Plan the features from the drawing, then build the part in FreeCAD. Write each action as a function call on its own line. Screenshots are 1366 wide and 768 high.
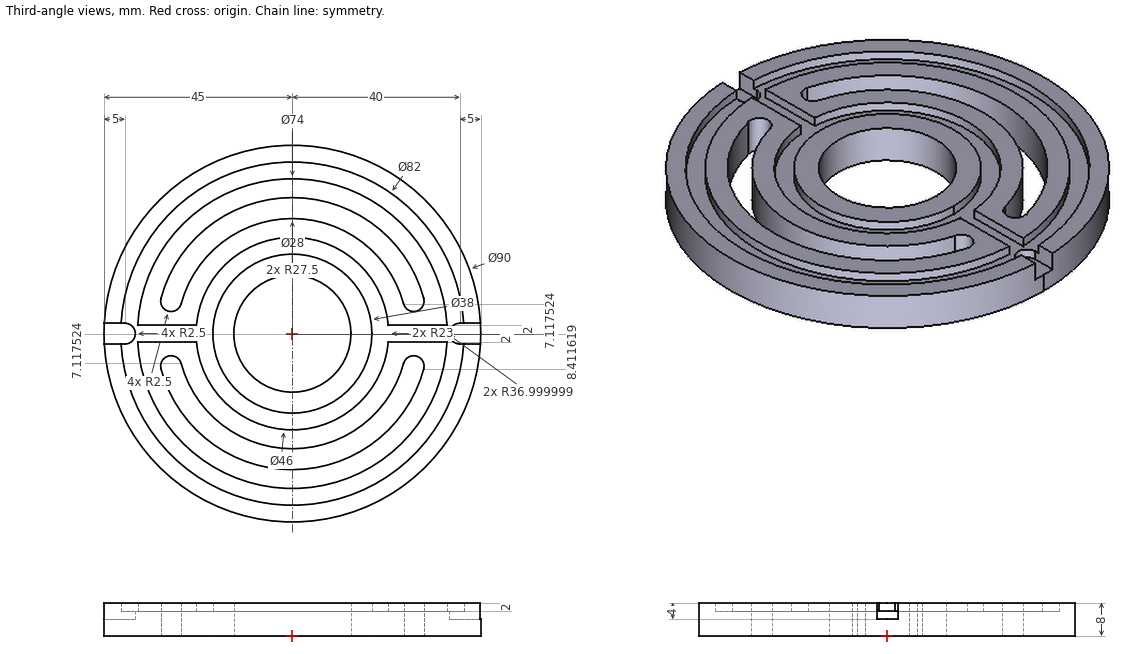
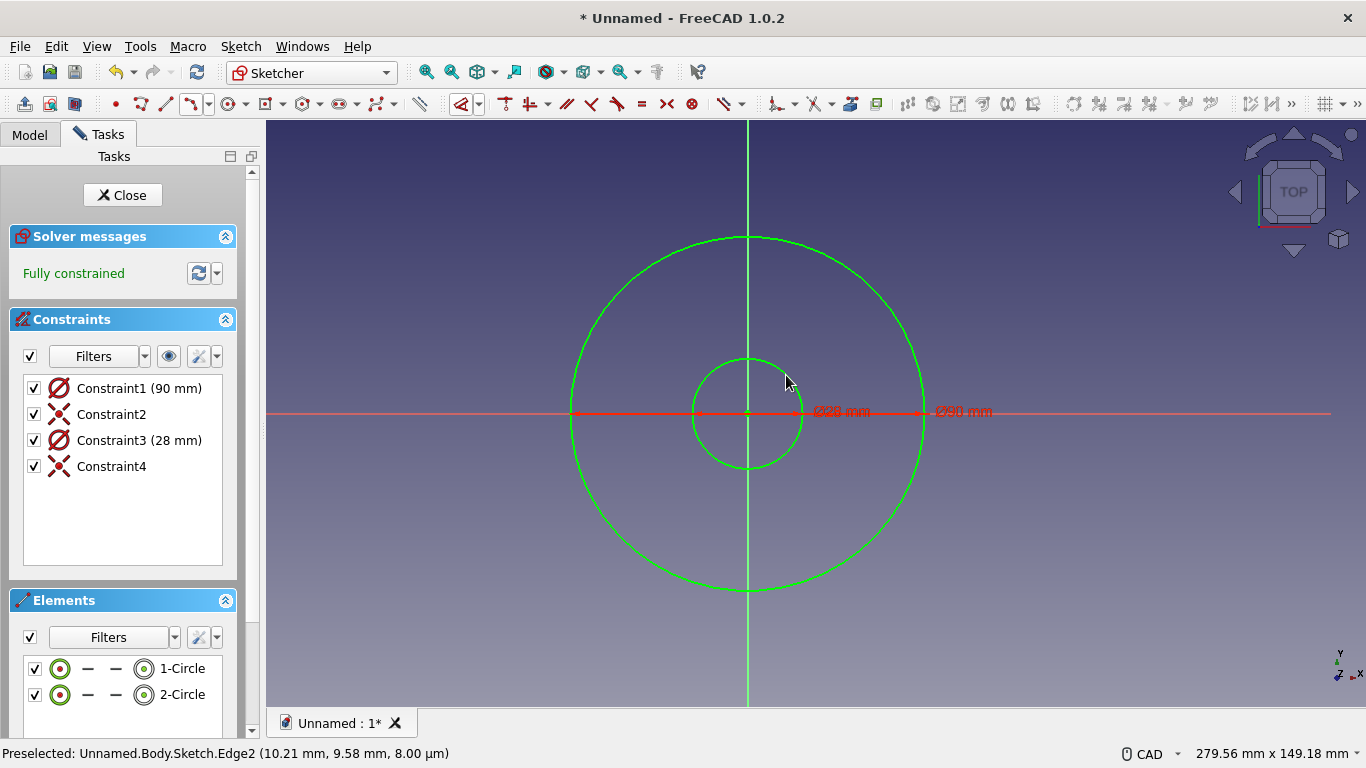
click(123, 195)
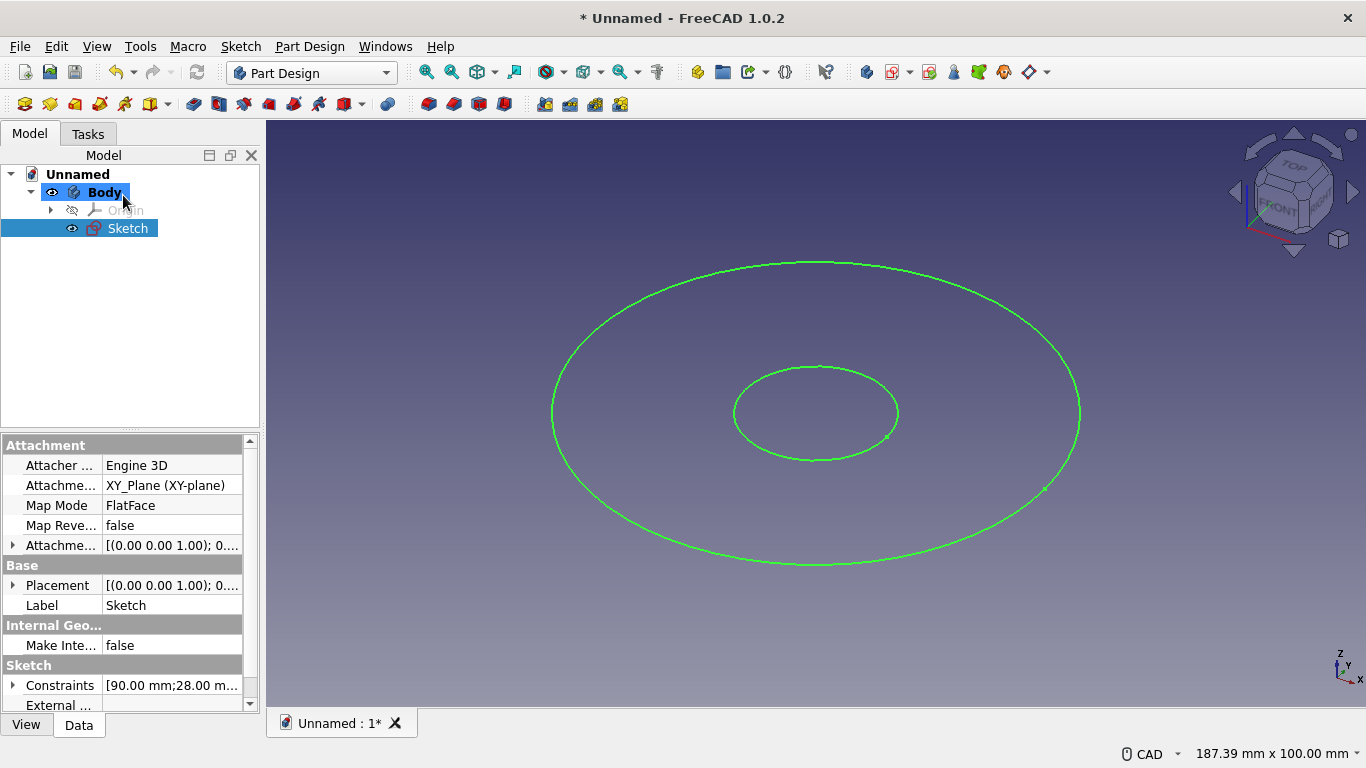
click(25, 104)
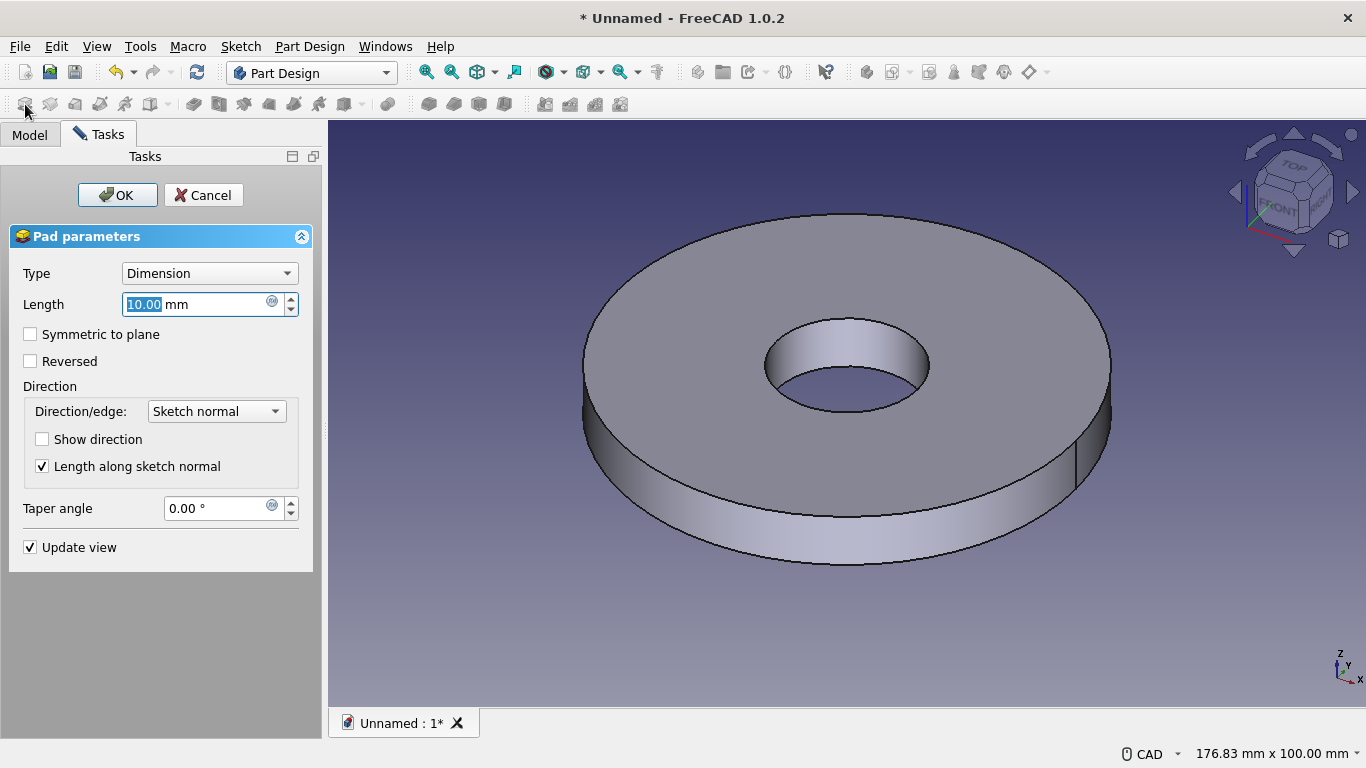
text(8)
key(Tab)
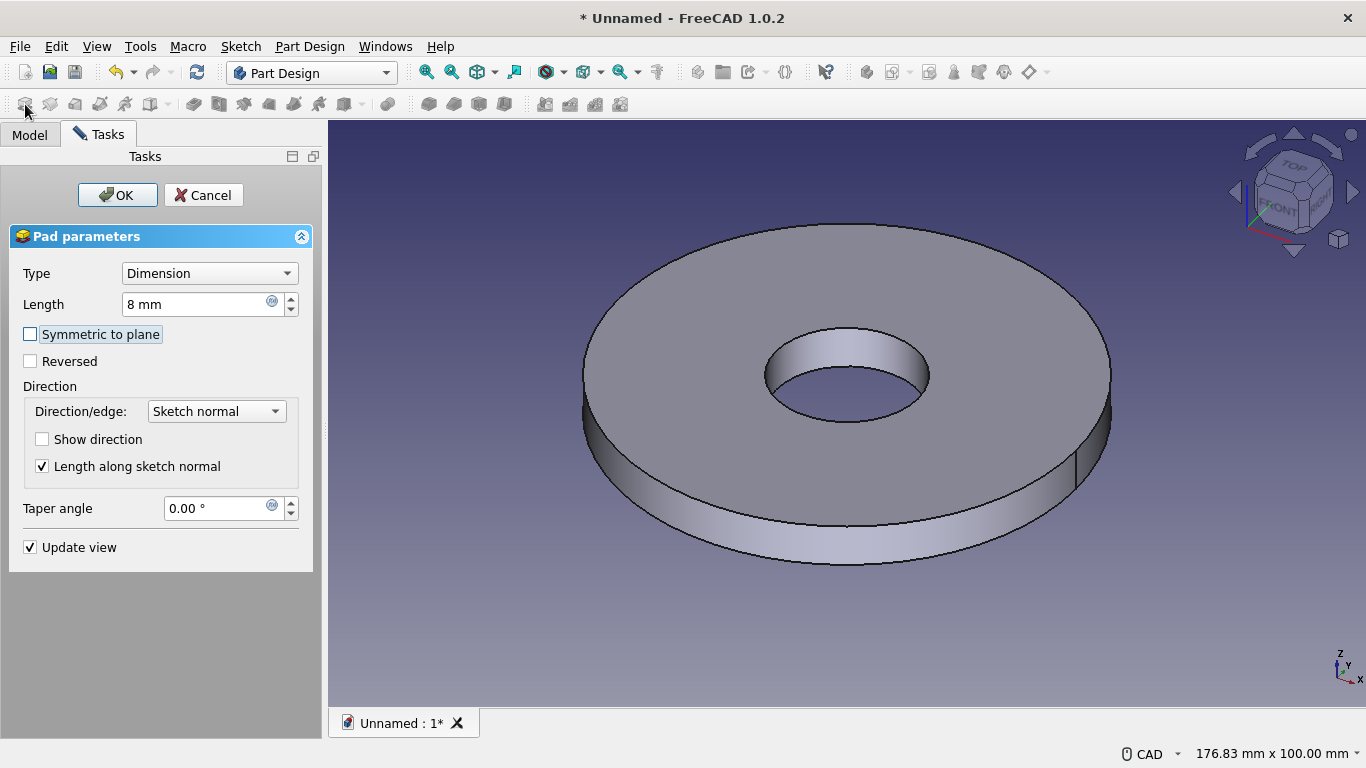
click(118, 195)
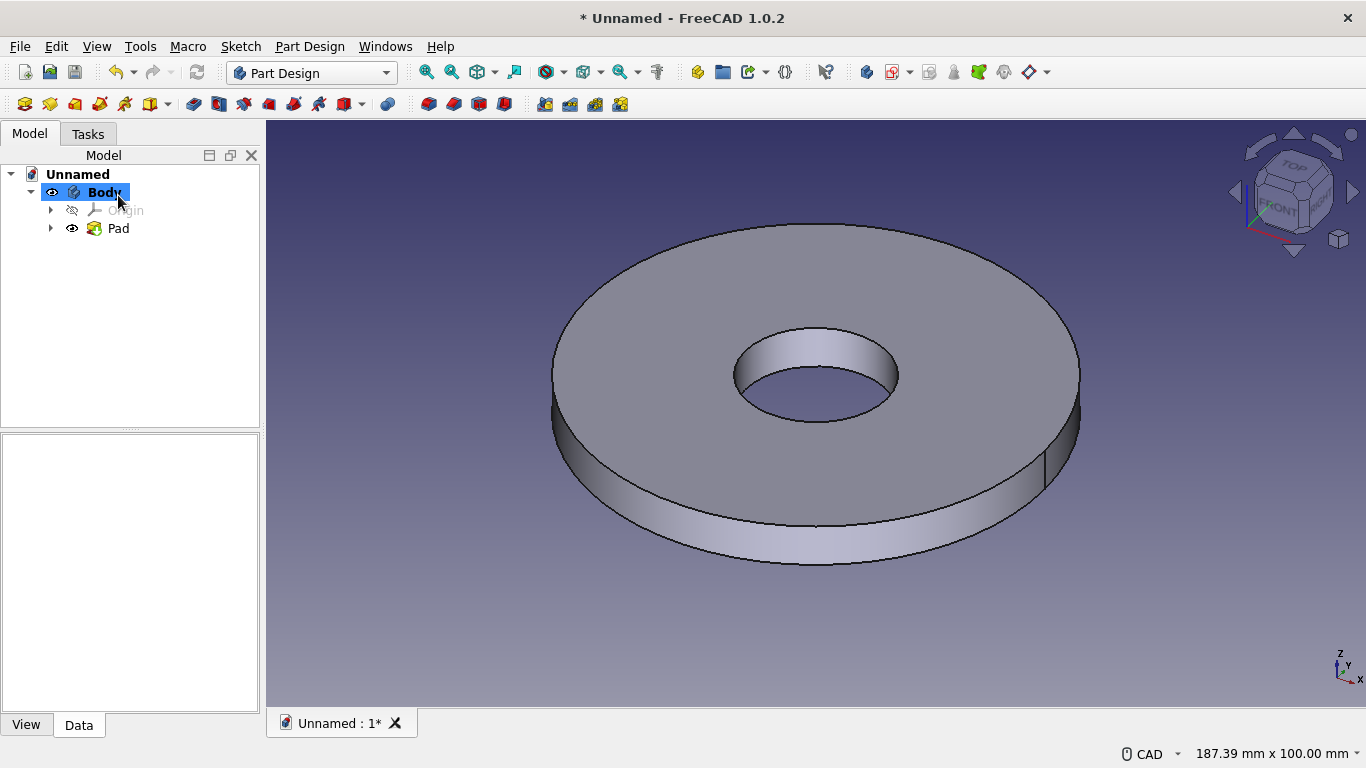
click(675, 427)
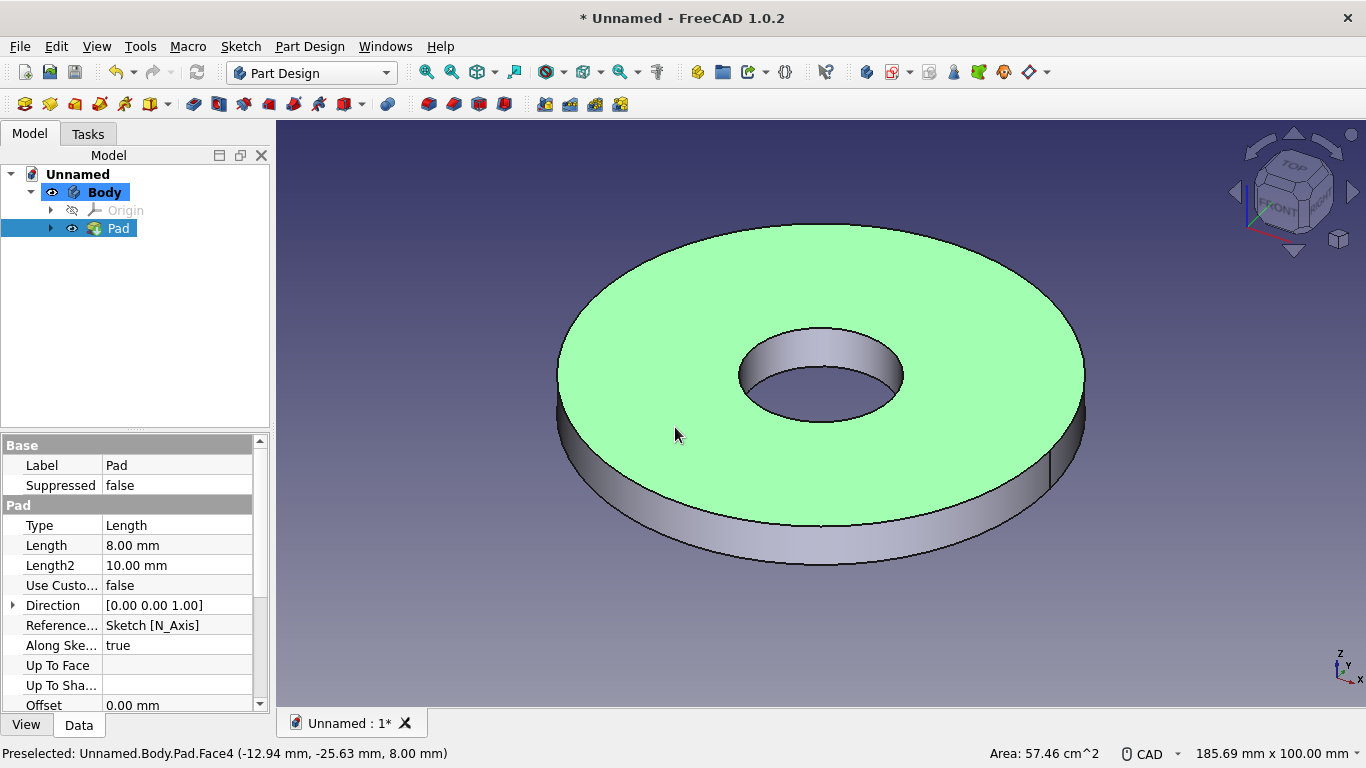
click(892, 72)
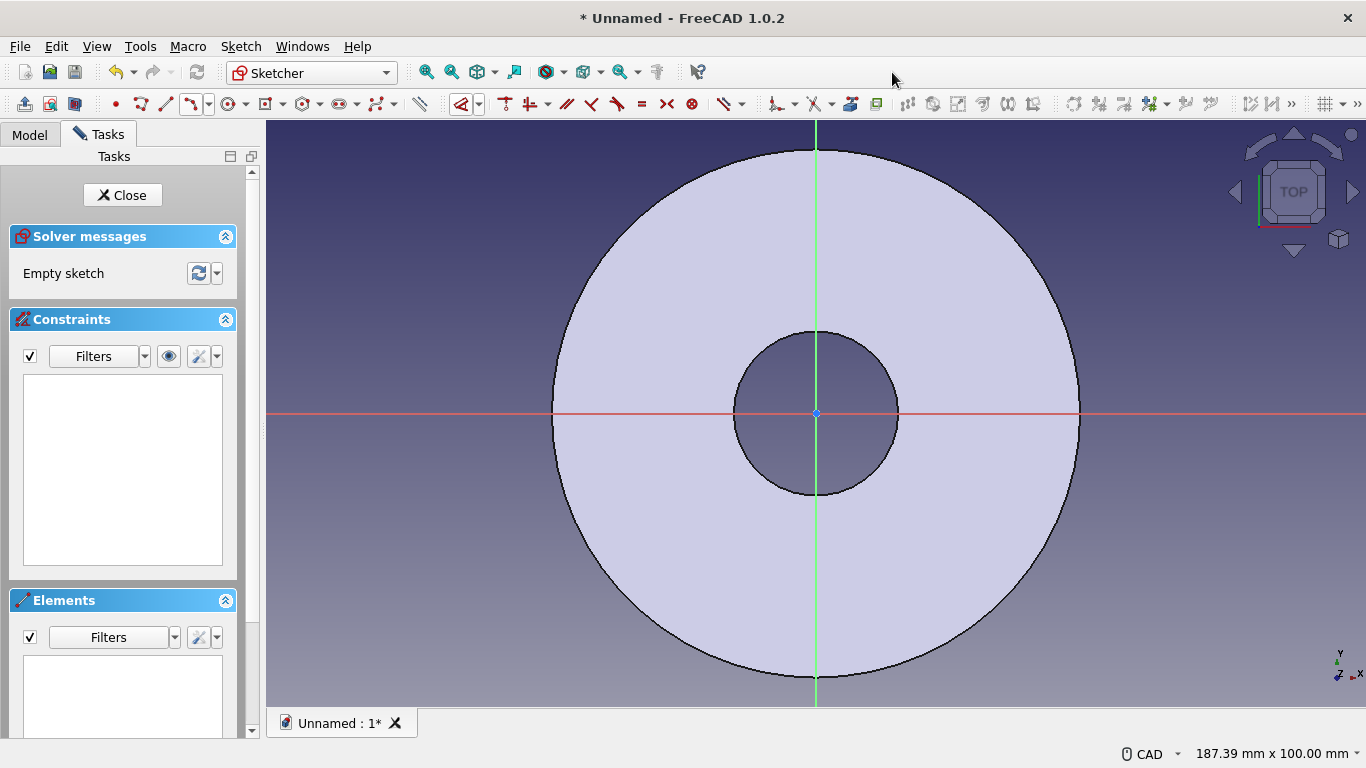
scroll(438, 413, down, 1)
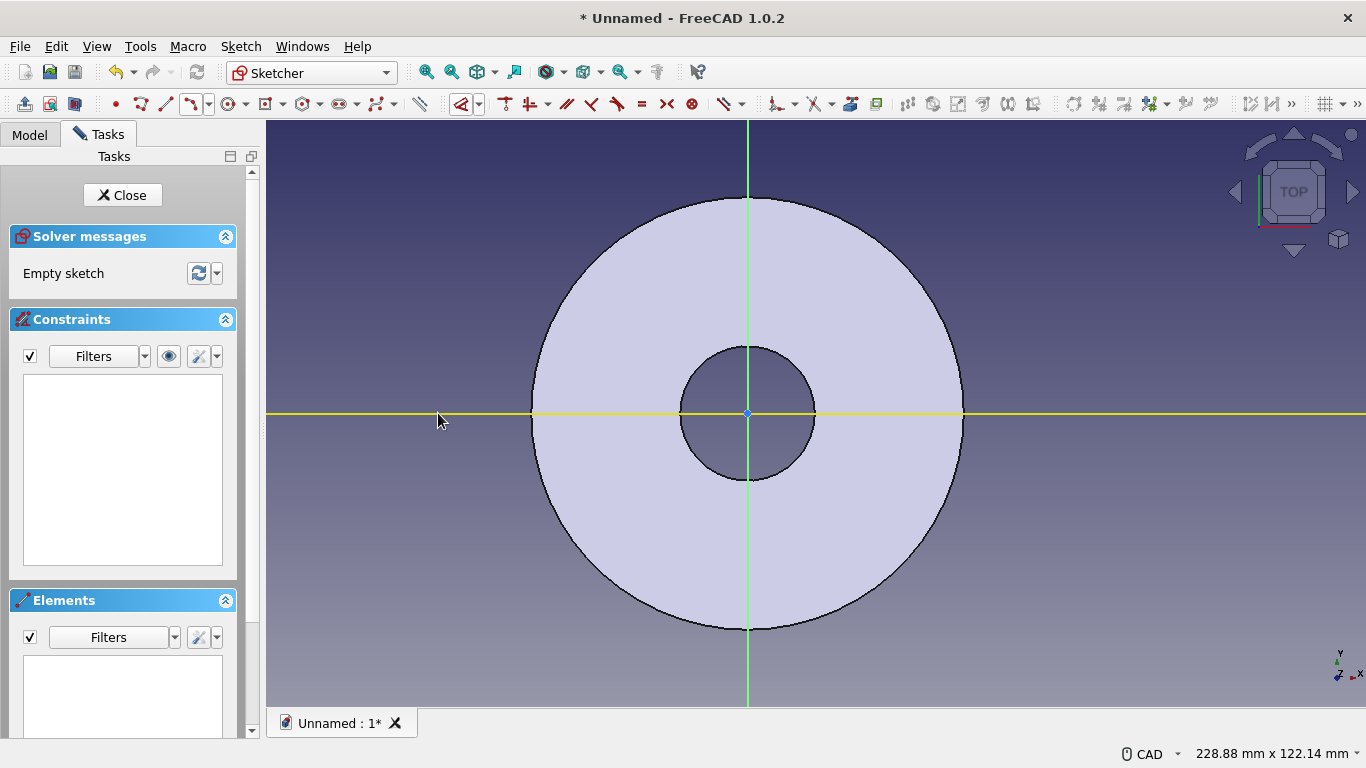
key(g)
key(3)
key(a)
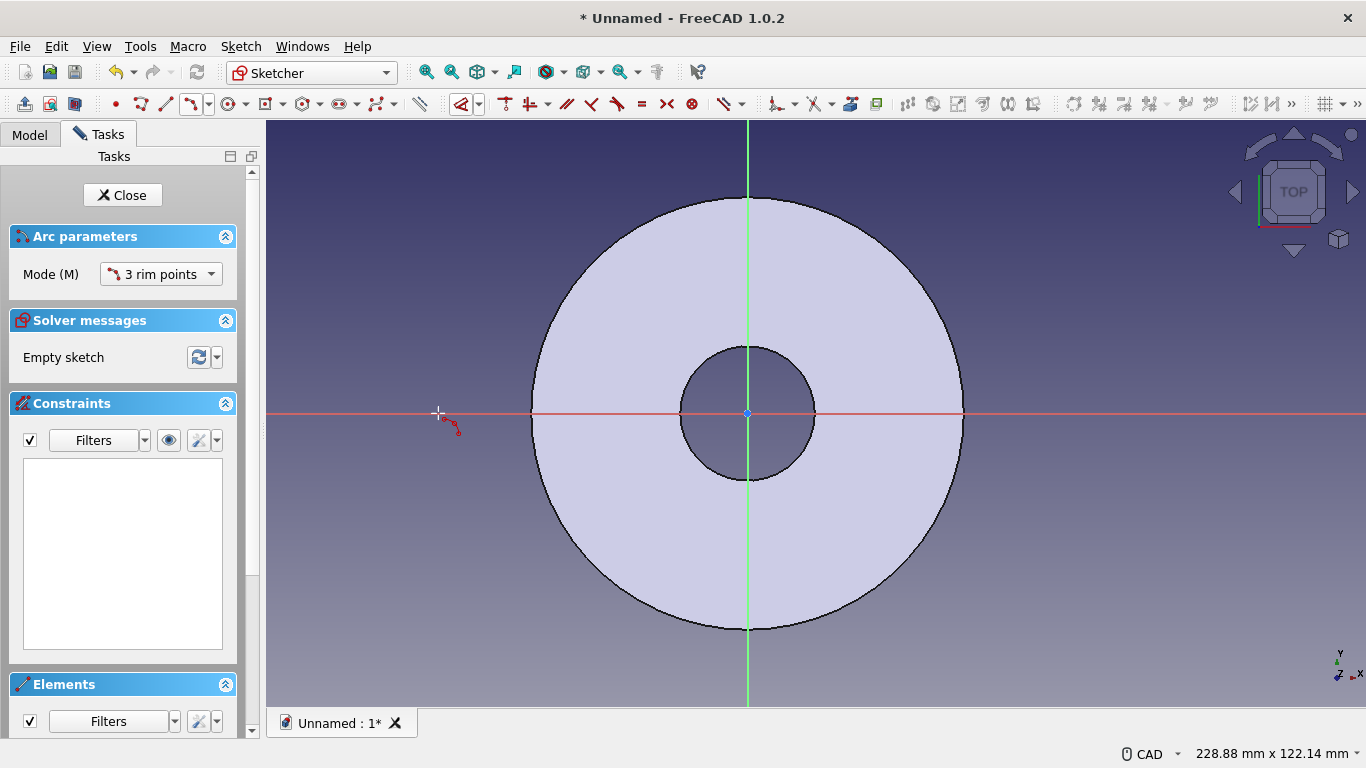
click(620, 379)
click(875, 379)
click(782, 286)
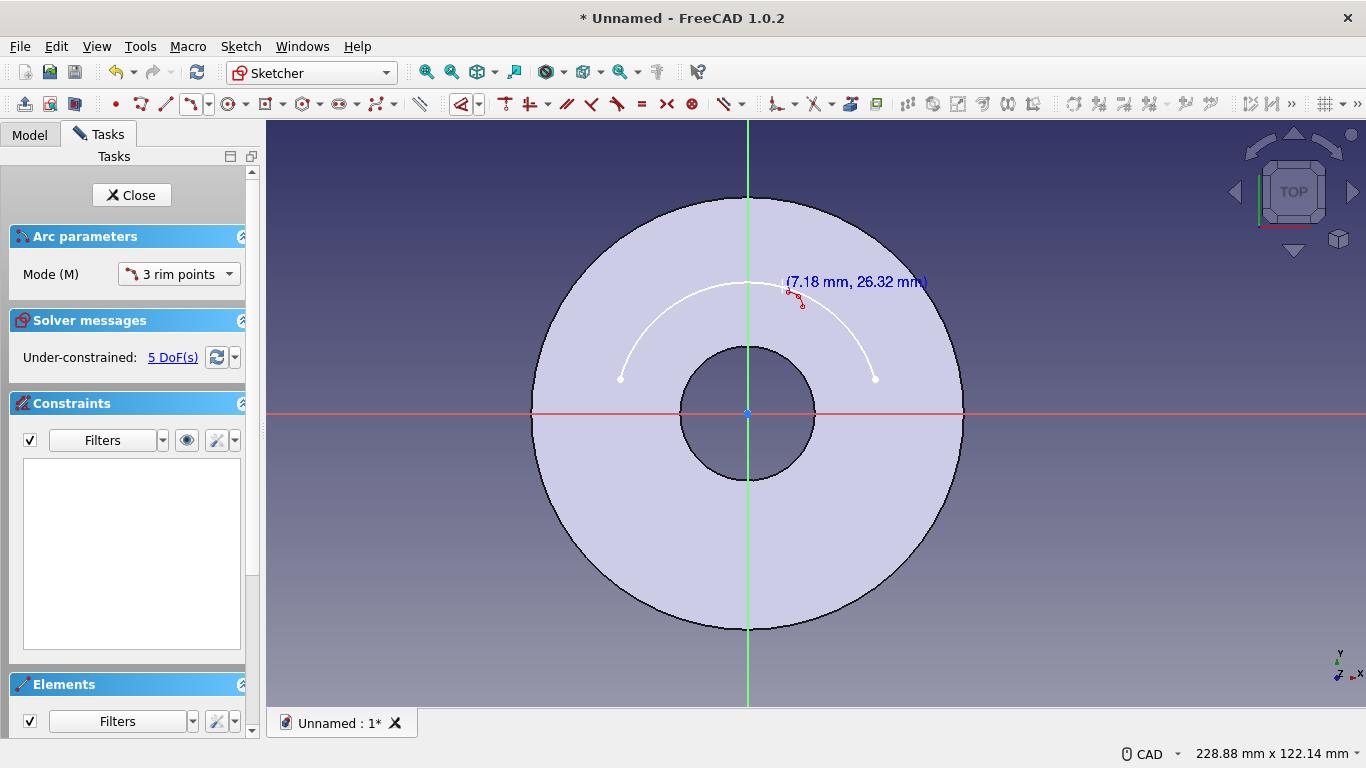
click(875, 380)
click(898, 373)